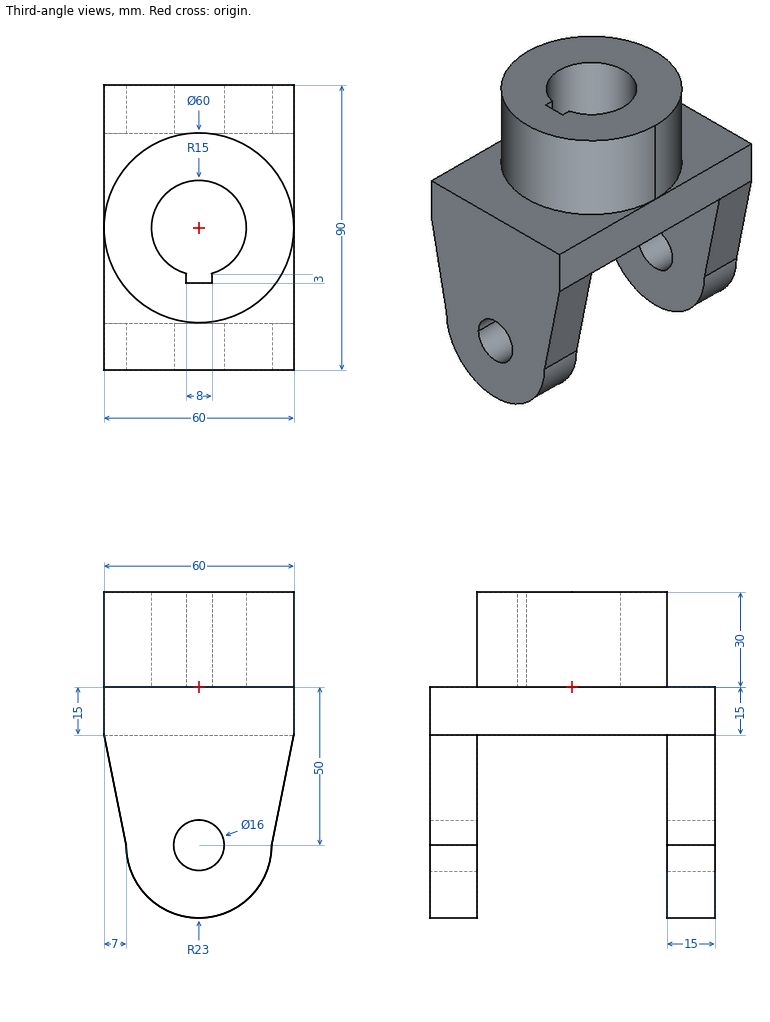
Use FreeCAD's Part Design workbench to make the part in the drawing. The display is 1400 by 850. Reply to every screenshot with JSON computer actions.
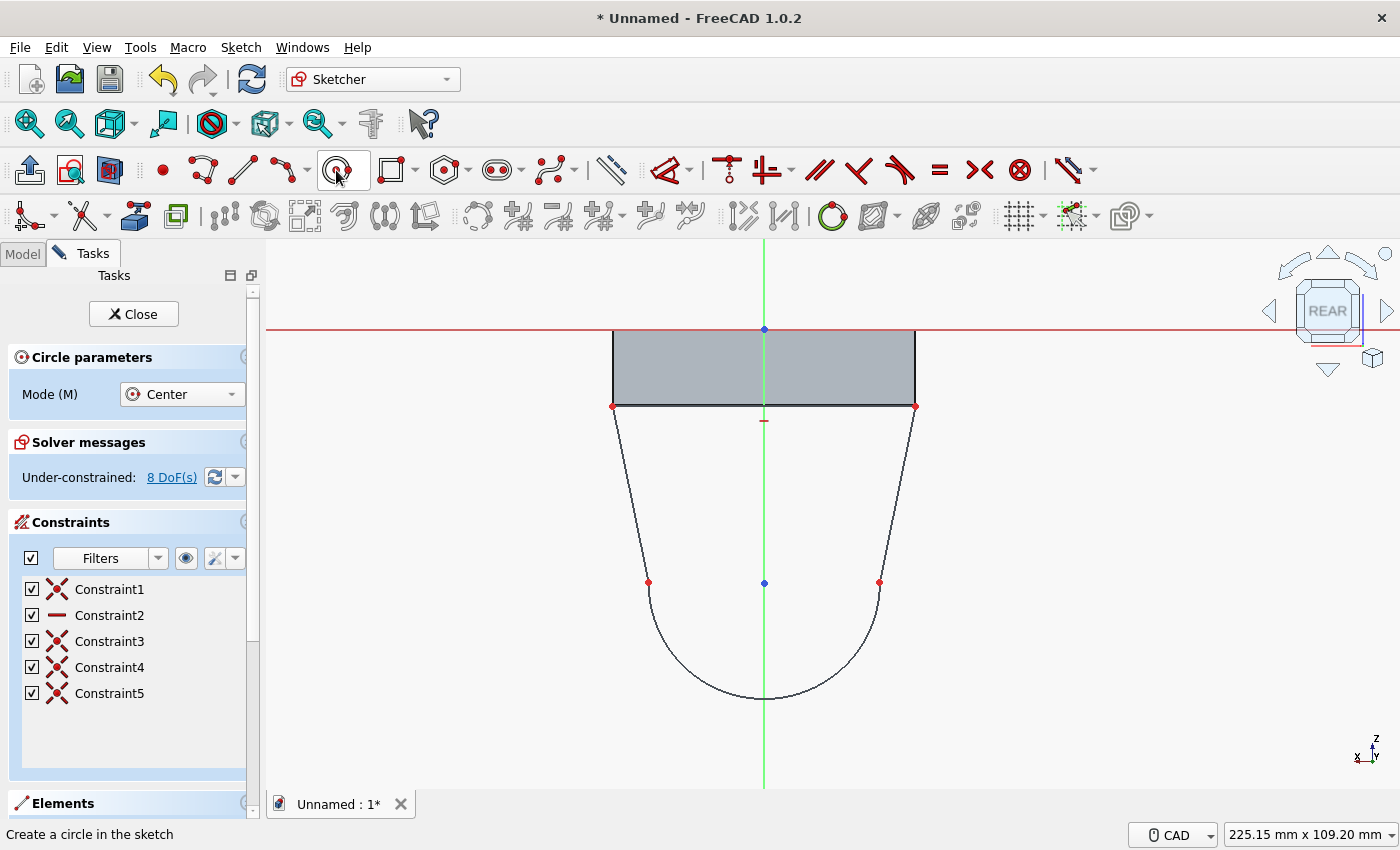
{"action": "left_click", "coordinate": [764, 582]}
{"action": "mouse_move", "coordinate": [793, 553]}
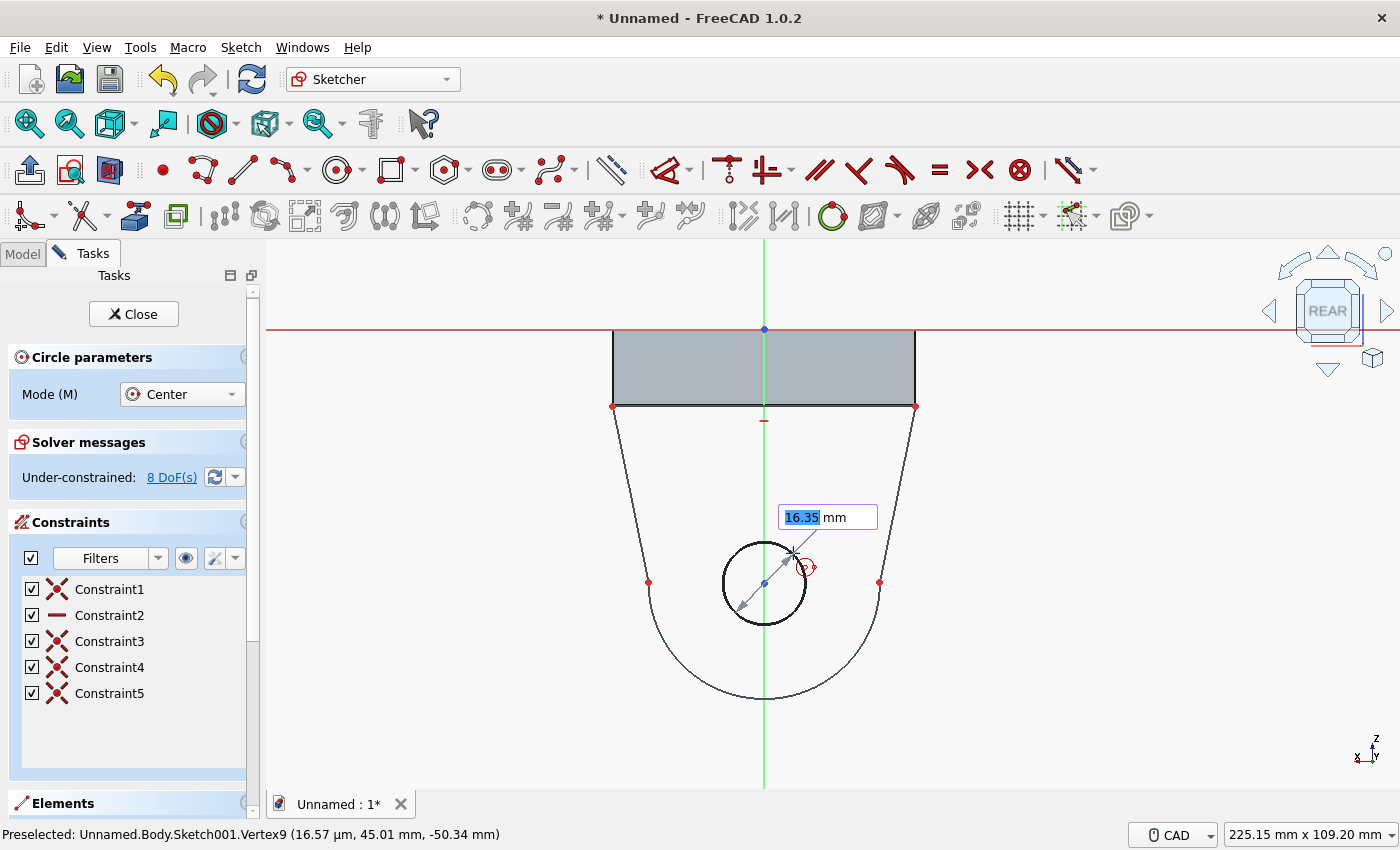
{"action": "type", "text": "16"}
{"action": "key", "text": "Return"}
{"action": "key", "text": "Escape"}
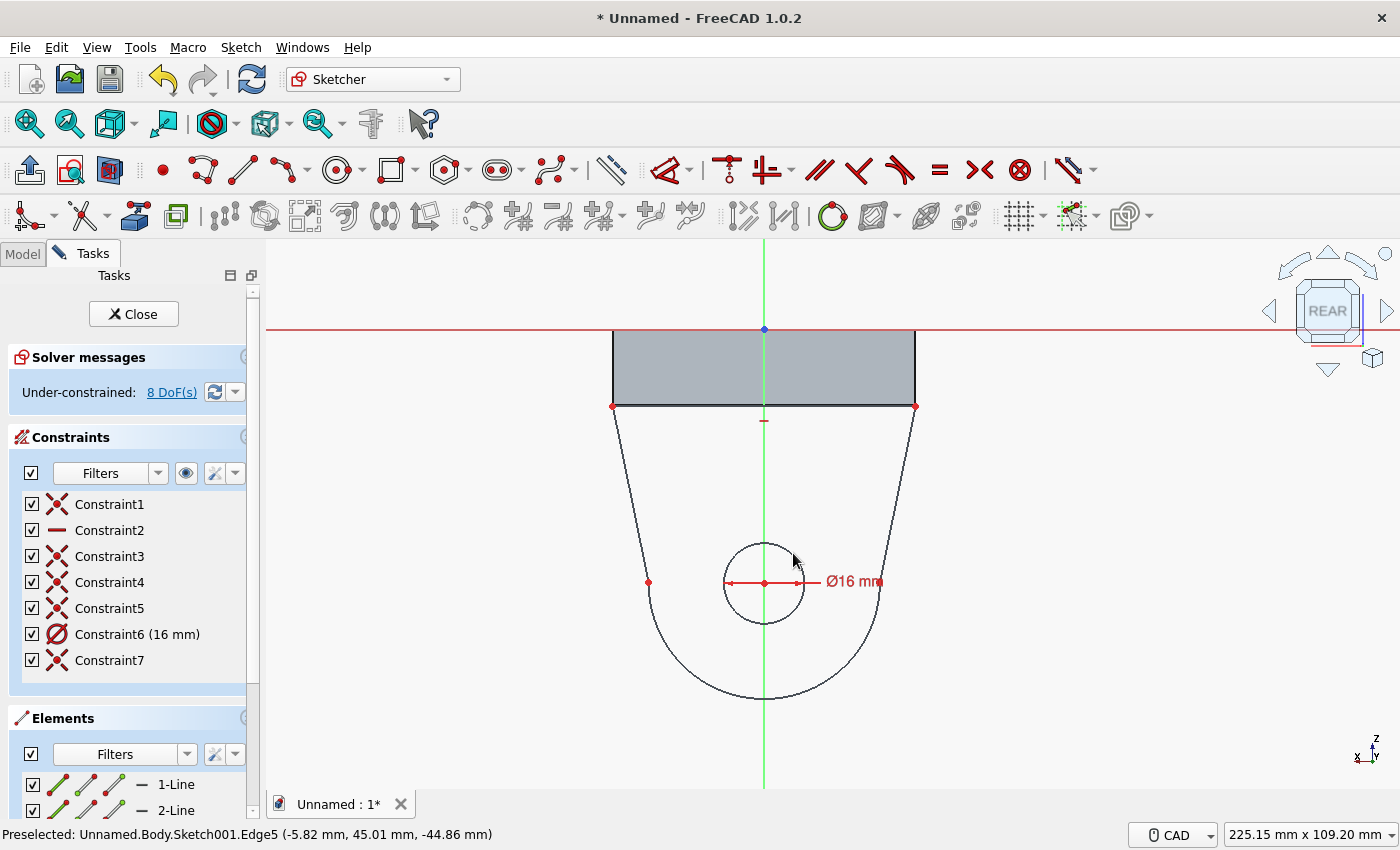
{"action": "left_click", "coordinate": [764, 583]}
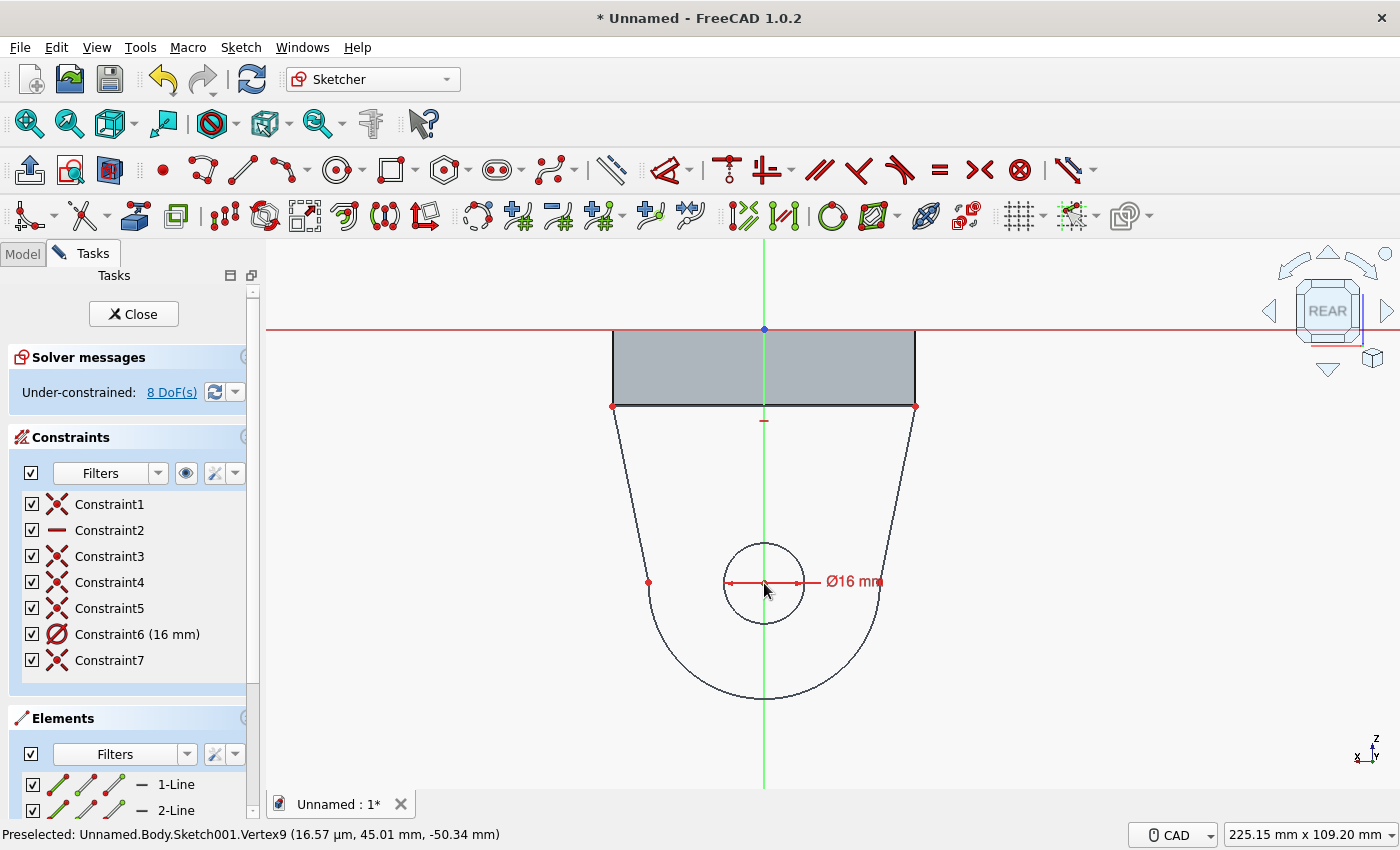
{"action": "left_click", "coordinate": [764, 655]}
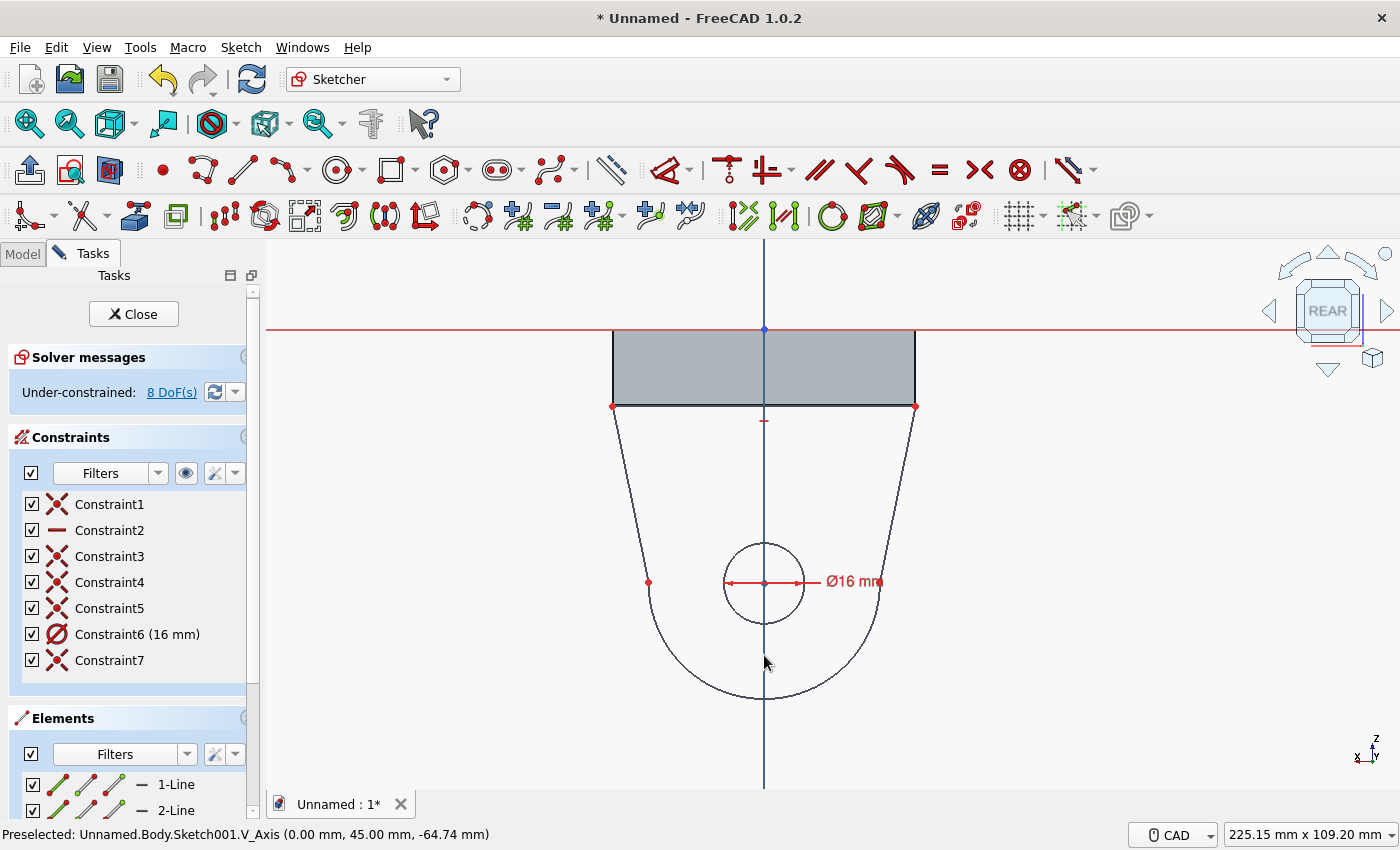
{"action": "left_click", "coordinate": [728, 170]}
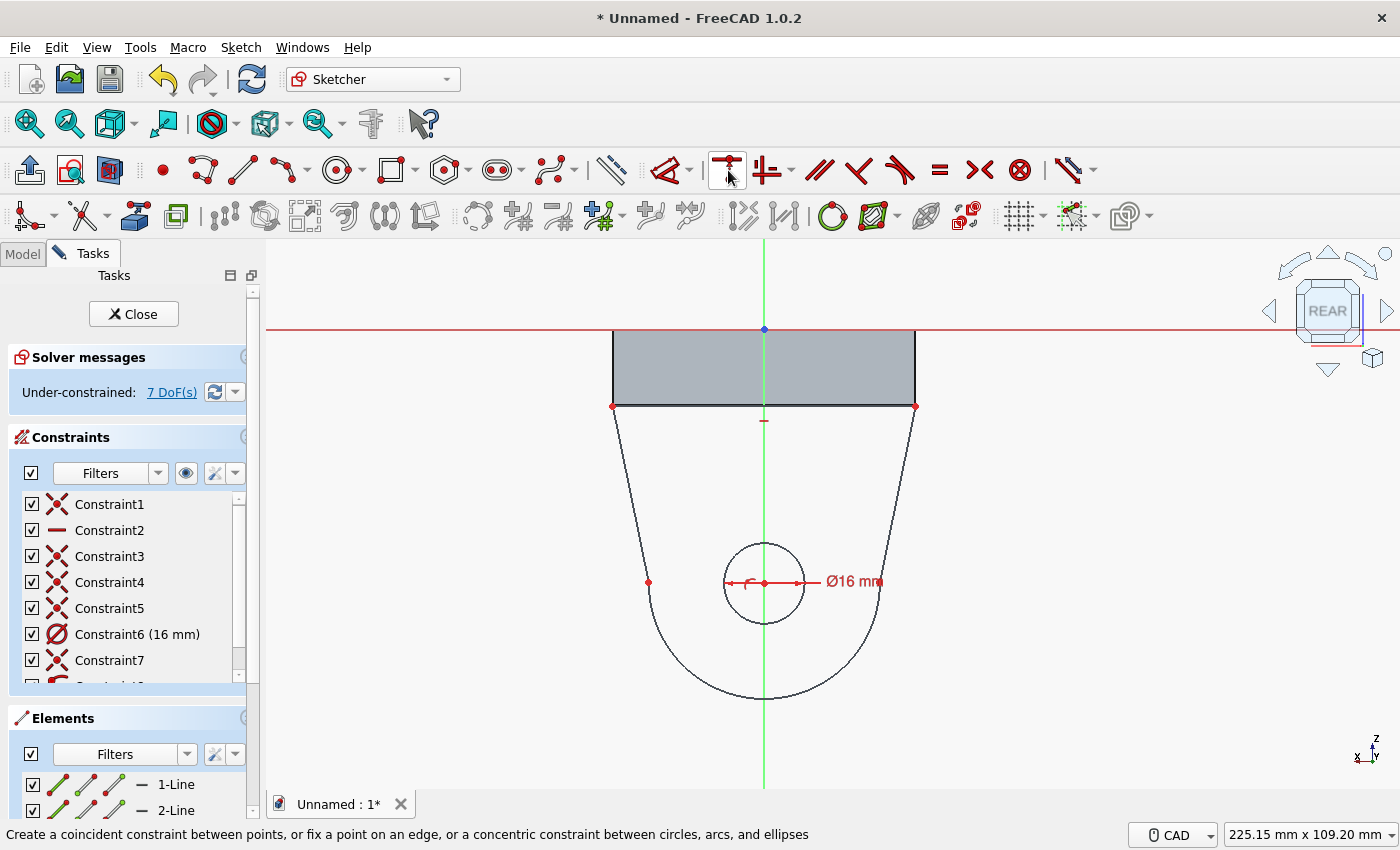
{"action": "left_click", "coordinate": [666, 170]}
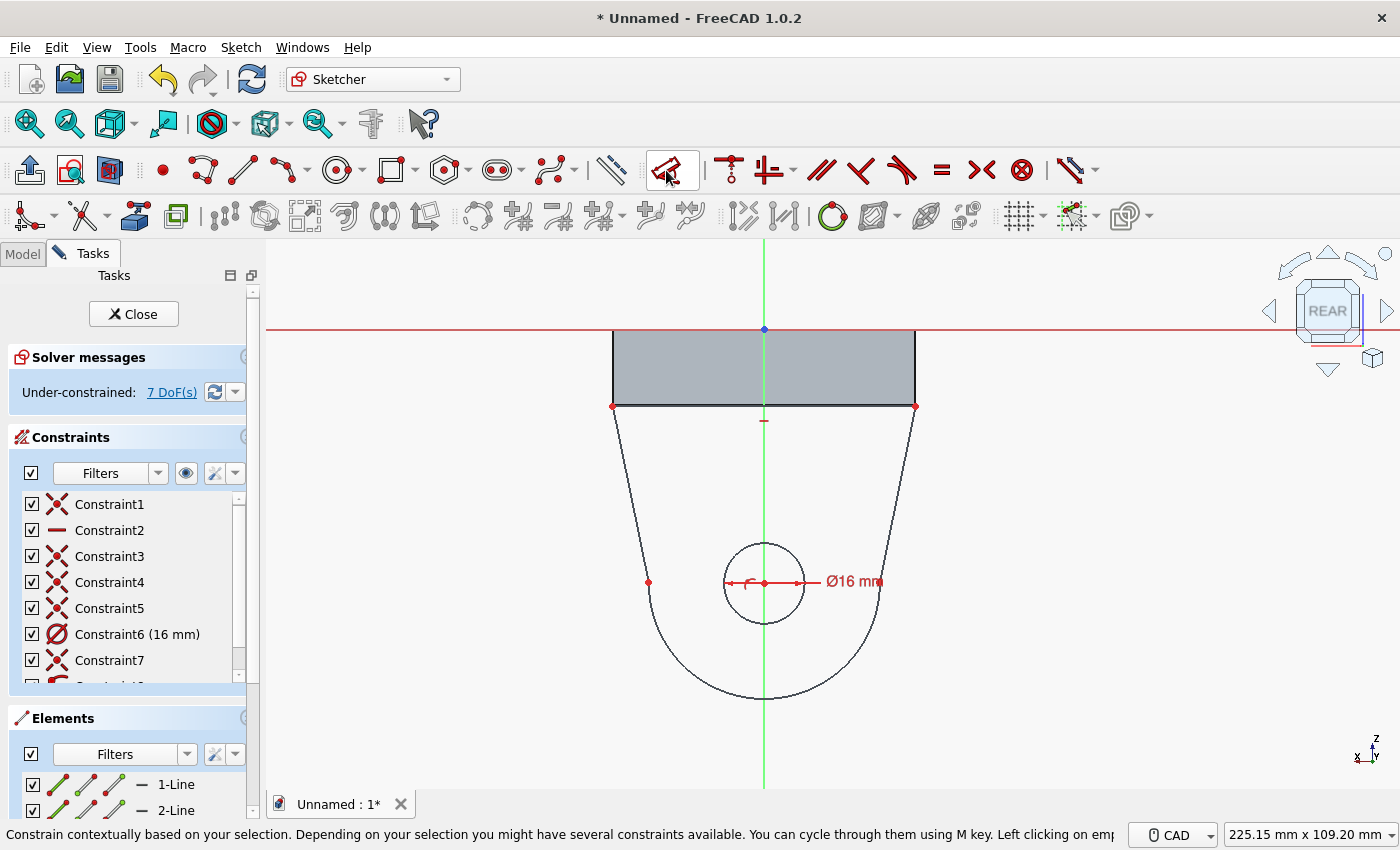
{"action": "left_click", "coordinate": [696, 677]}
{"action": "left_click", "coordinate": [677, 703]}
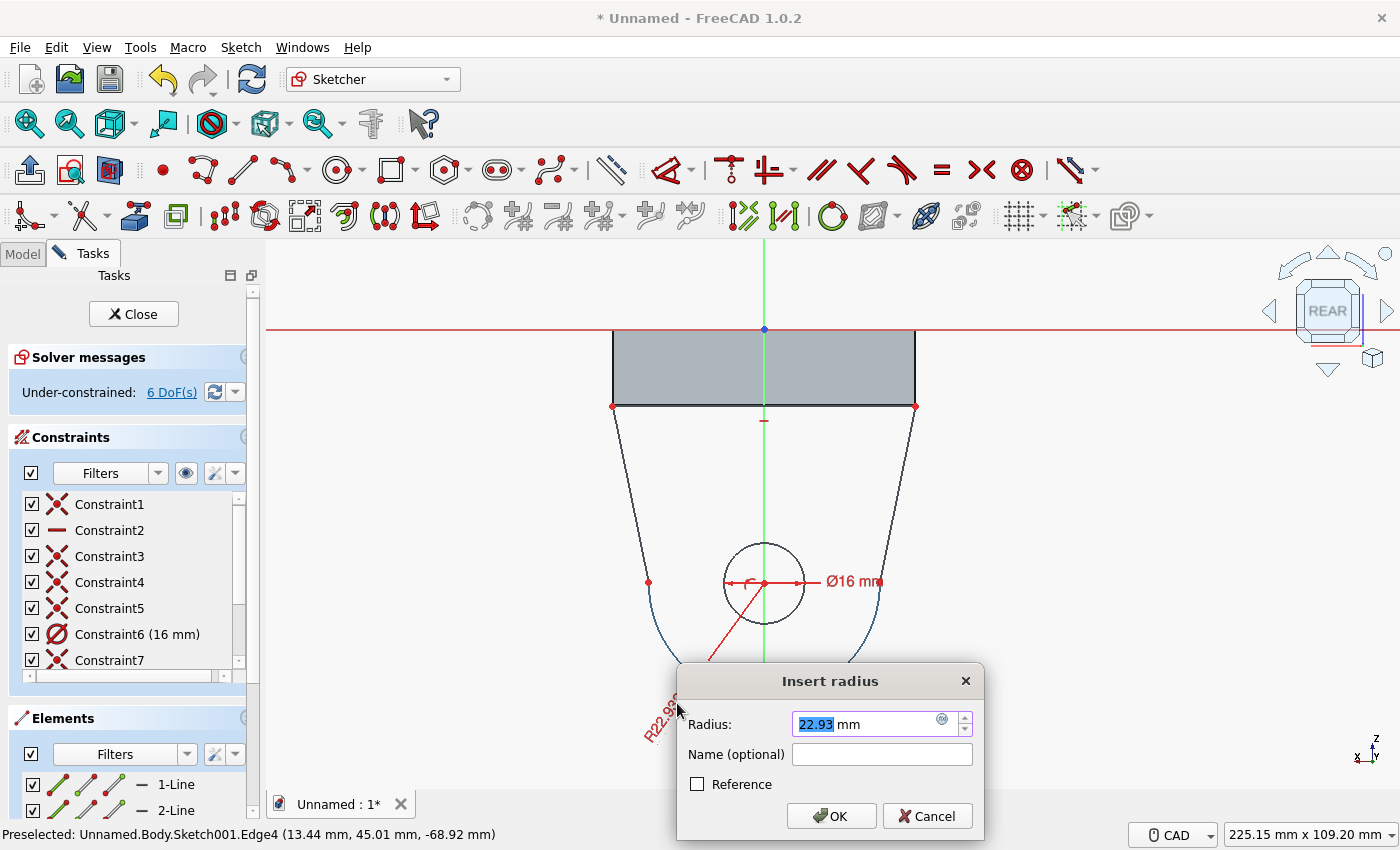
{"action": "type", "text": "23"}
{"action": "key", "text": "Return"}